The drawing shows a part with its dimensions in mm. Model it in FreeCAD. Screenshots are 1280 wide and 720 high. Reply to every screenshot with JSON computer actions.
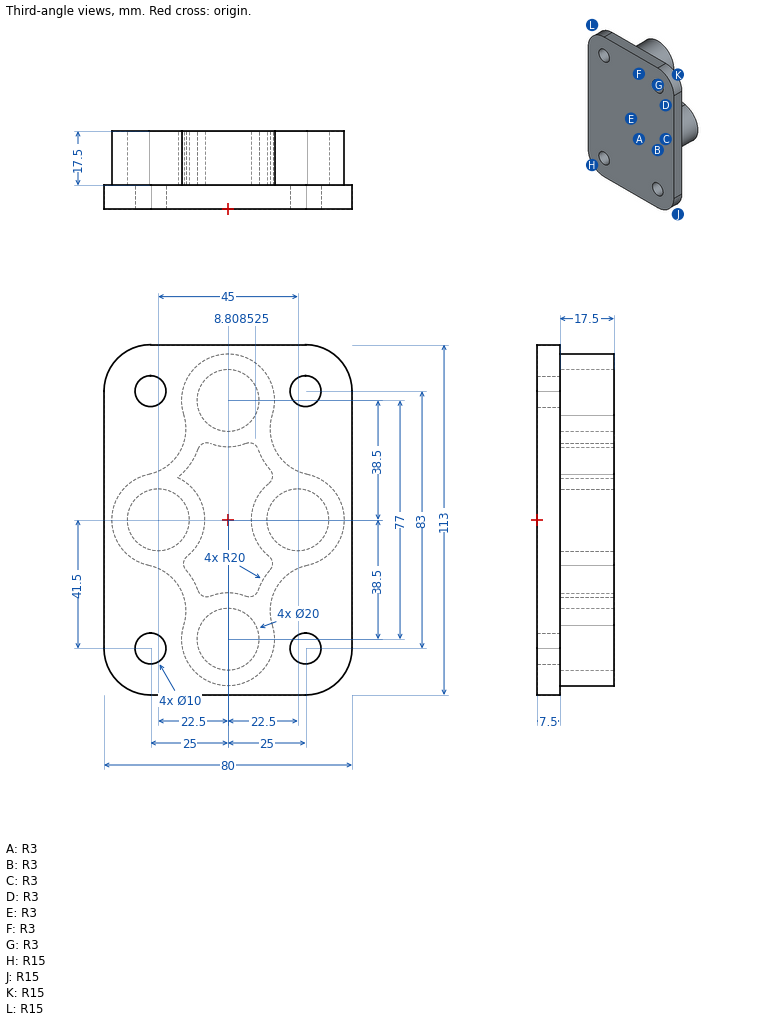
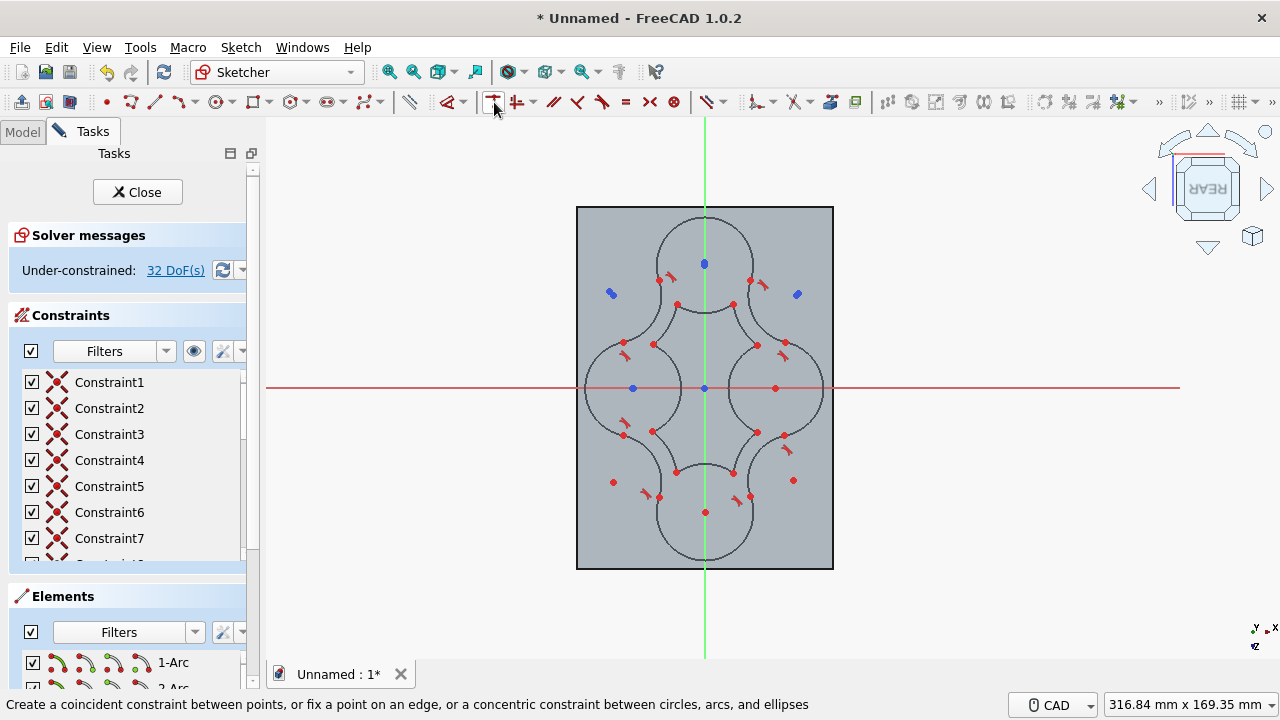
{"action": "left_click", "coordinate": [592, 364]}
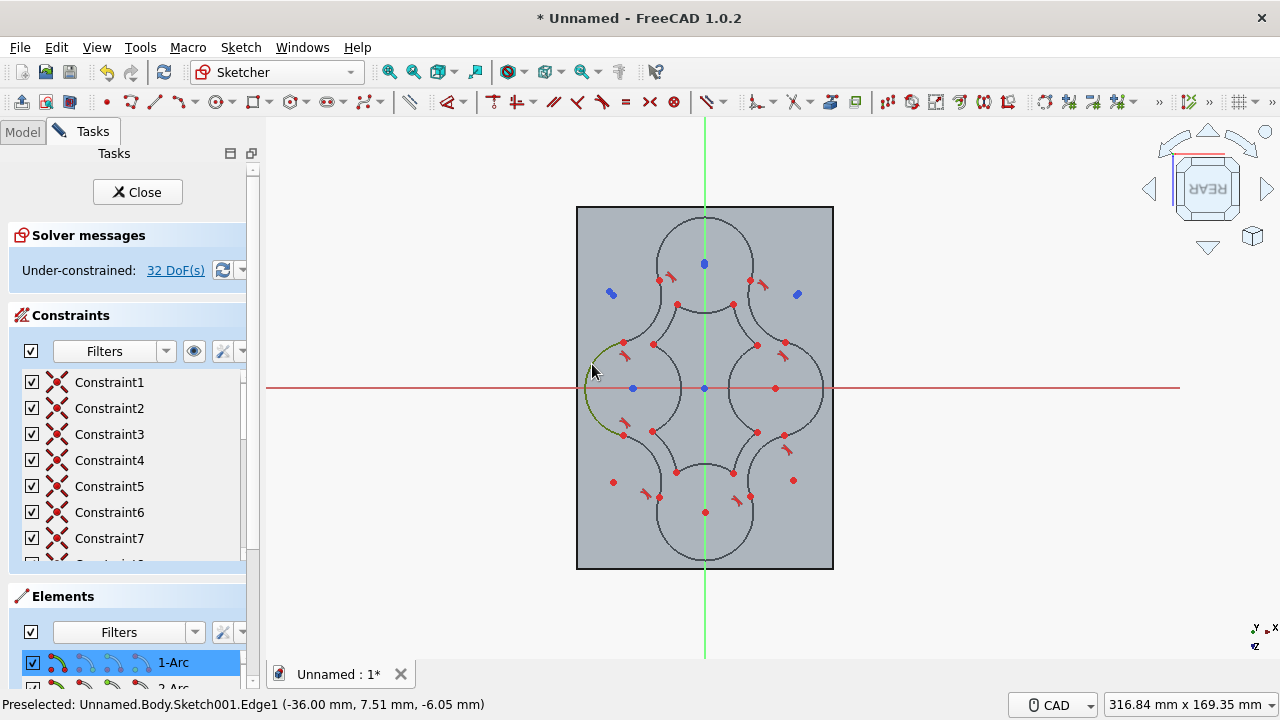
{"action": "left_click", "coordinate": [676, 410]}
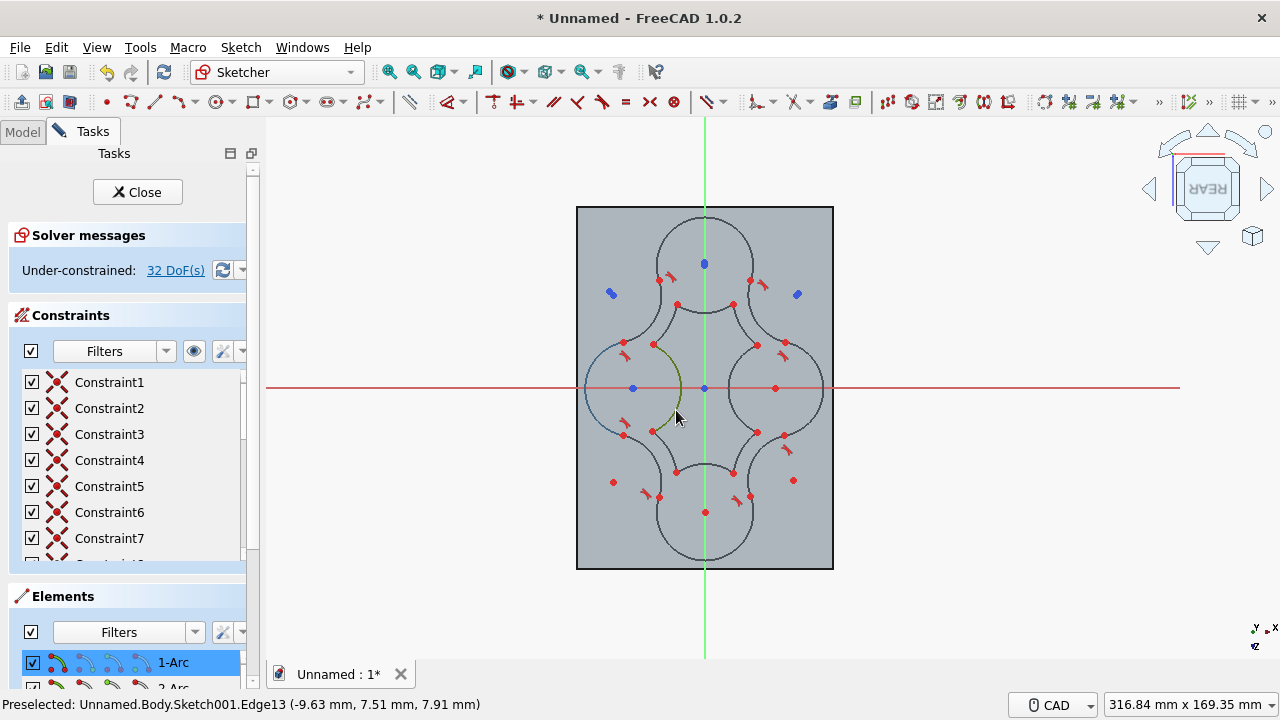
{"action": "left_click", "coordinate": [494, 102]}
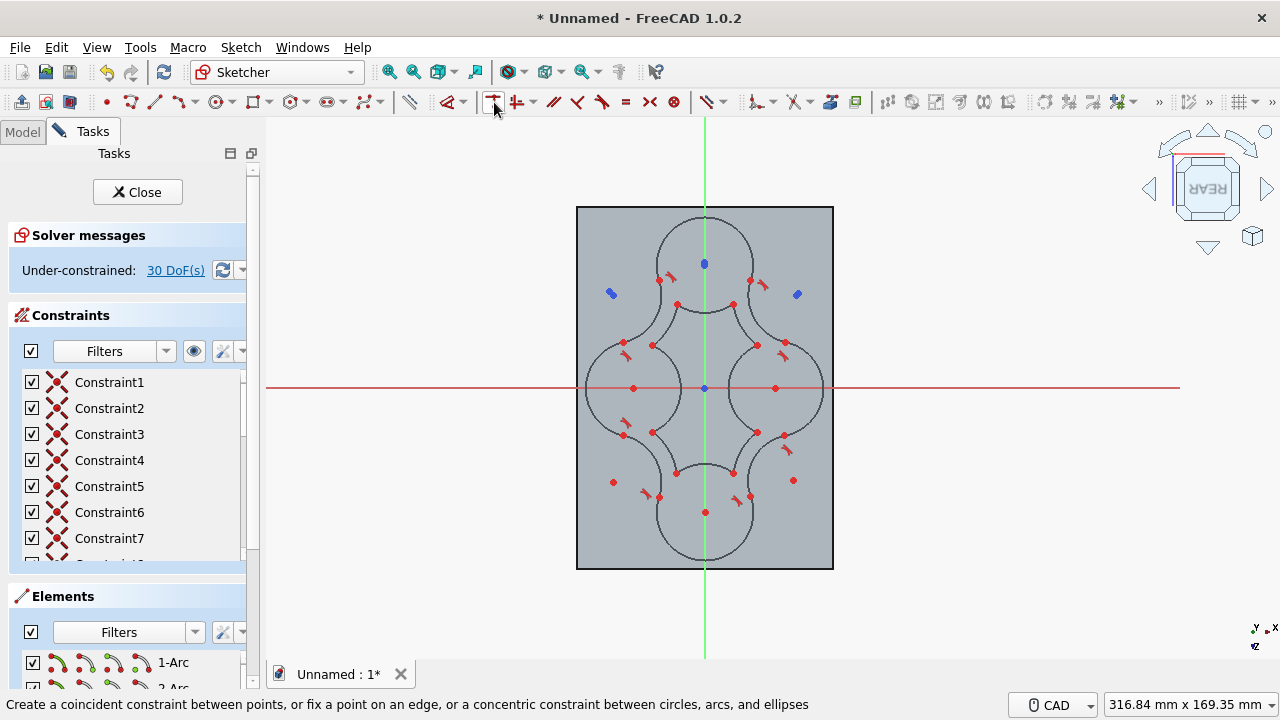
{"action": "left_click", "coordinate": [645, 332]}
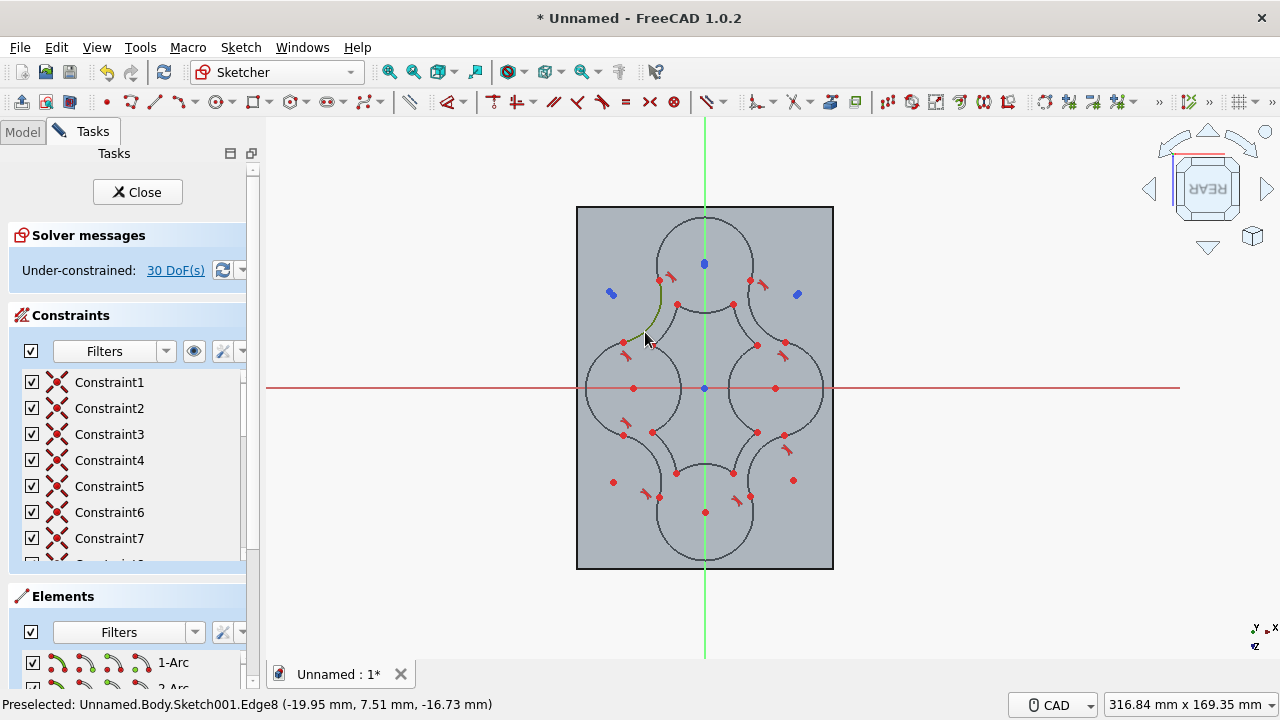
{"action": "left_click", "coordinate": [663, 336]}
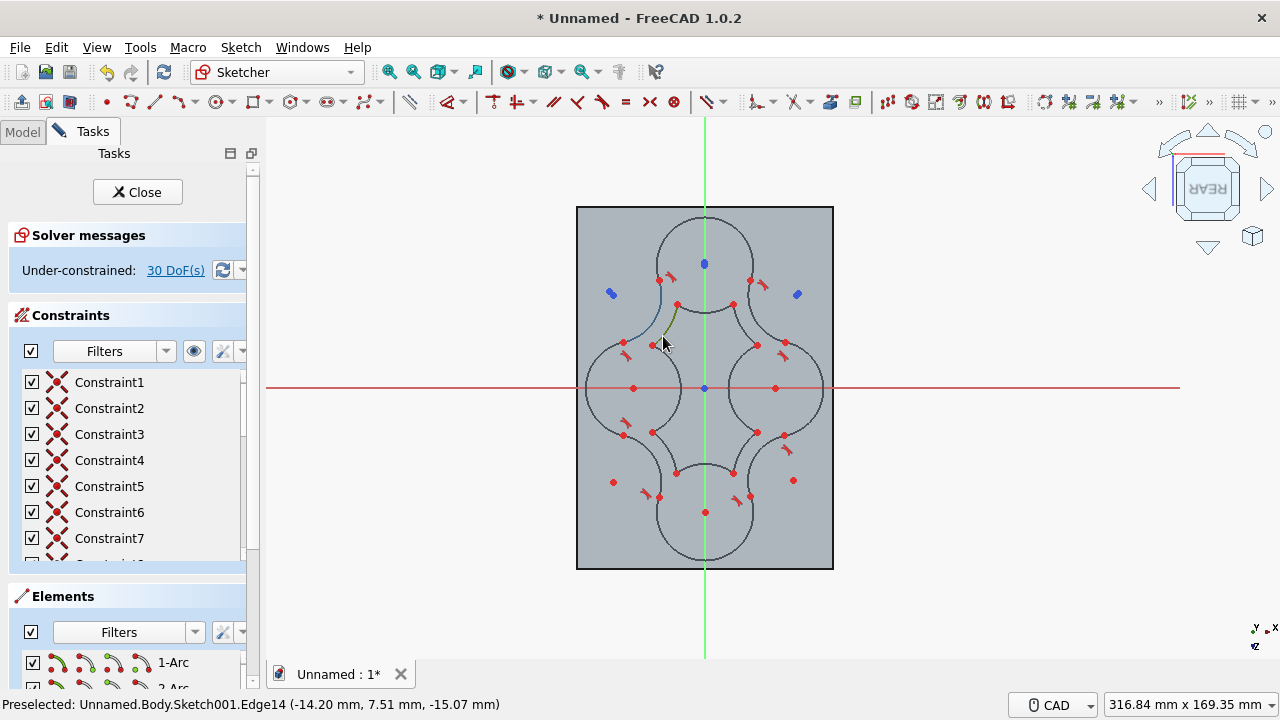
{"action": "key", "text": "c"}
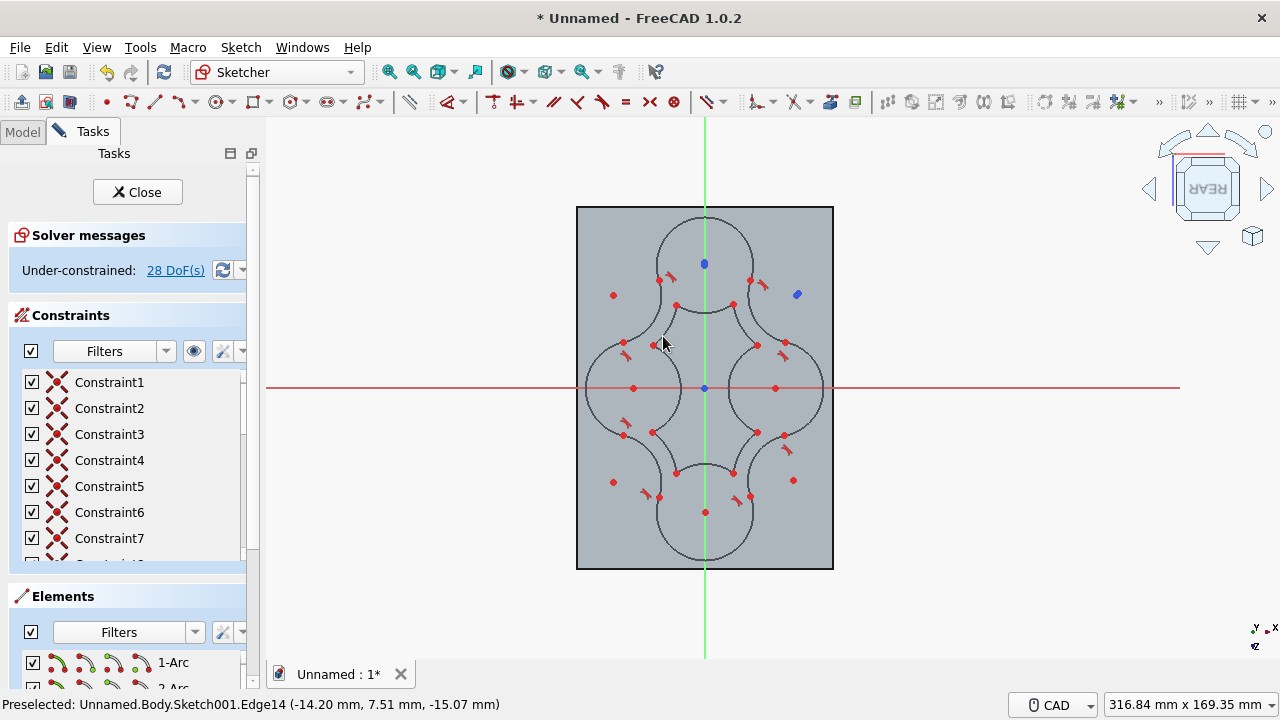
{"action": "left_click", "coordinate": [738, 231]}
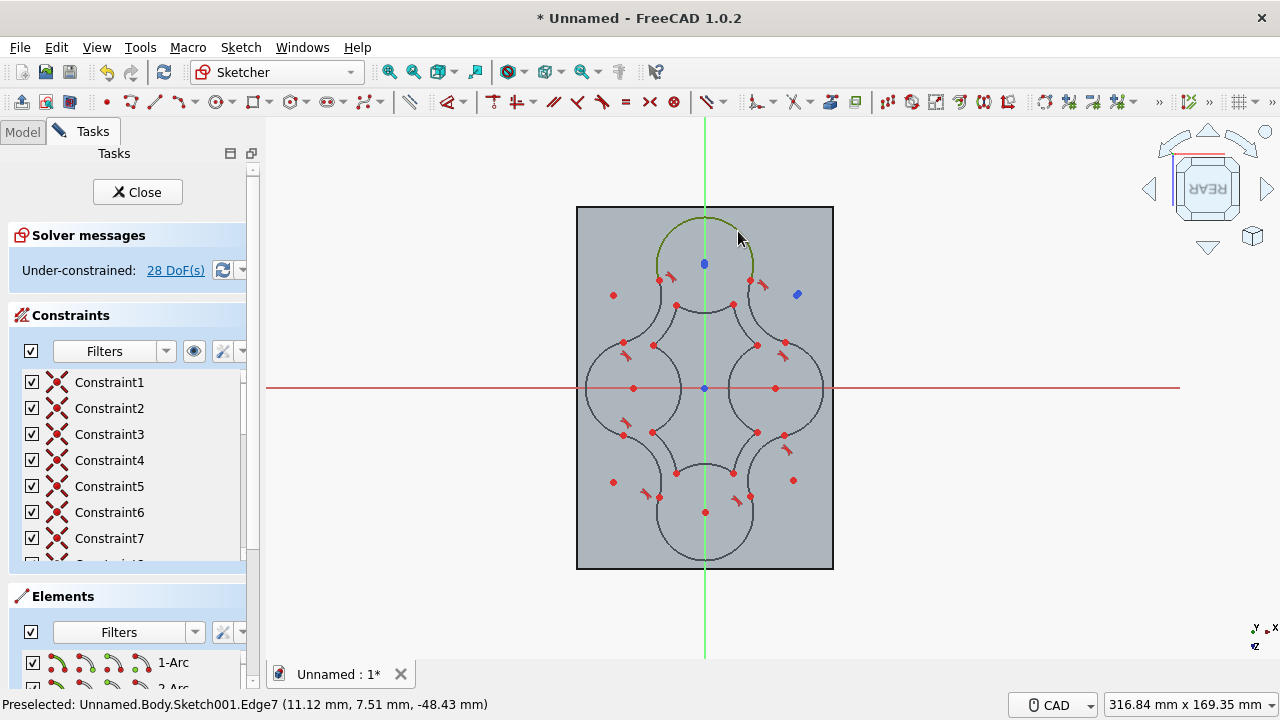
{"action": "left_click", "coordinate": [693, 312]}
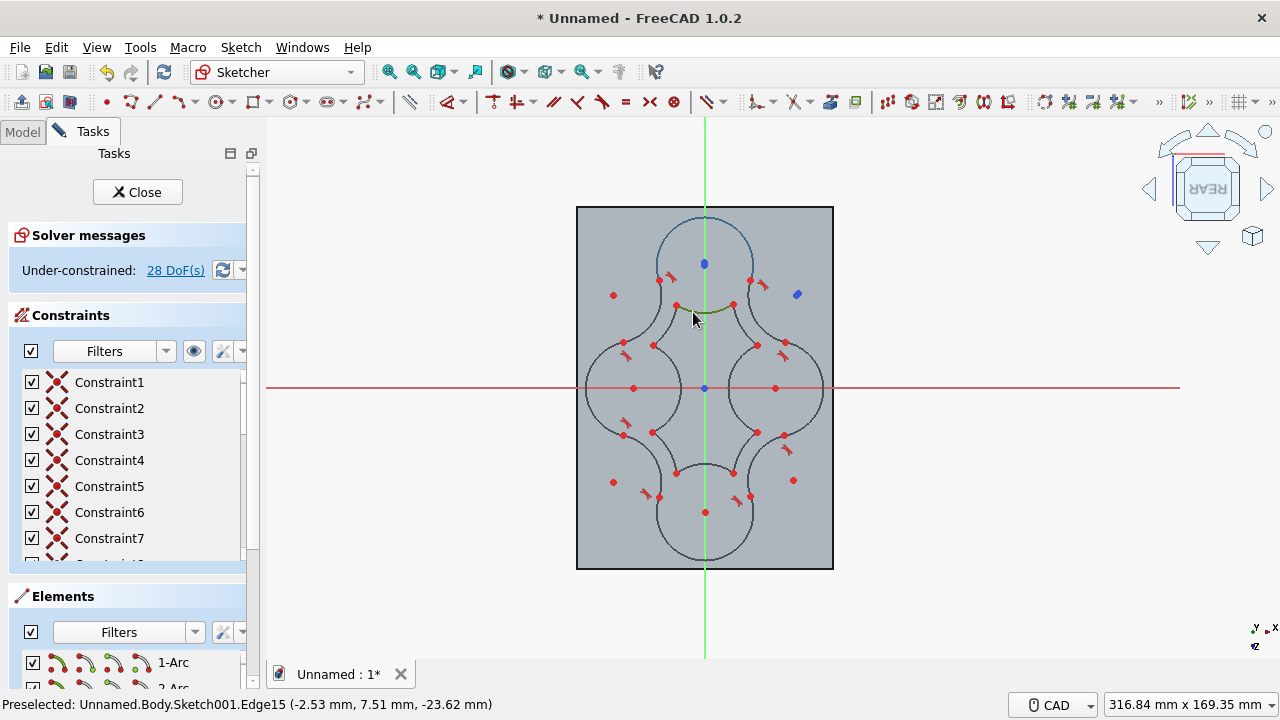
{"action": "left_click", "coordinate": [494, 102]}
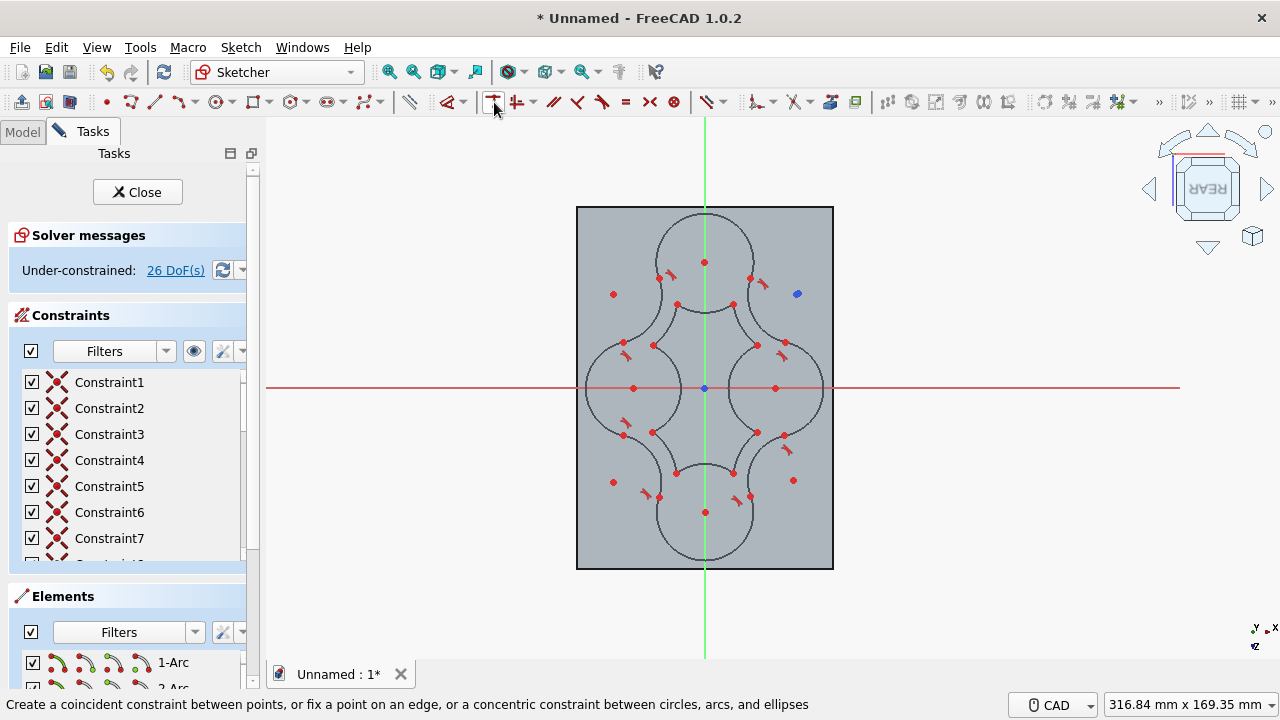
{"action": "left_click", "coordinate": [749, 303]}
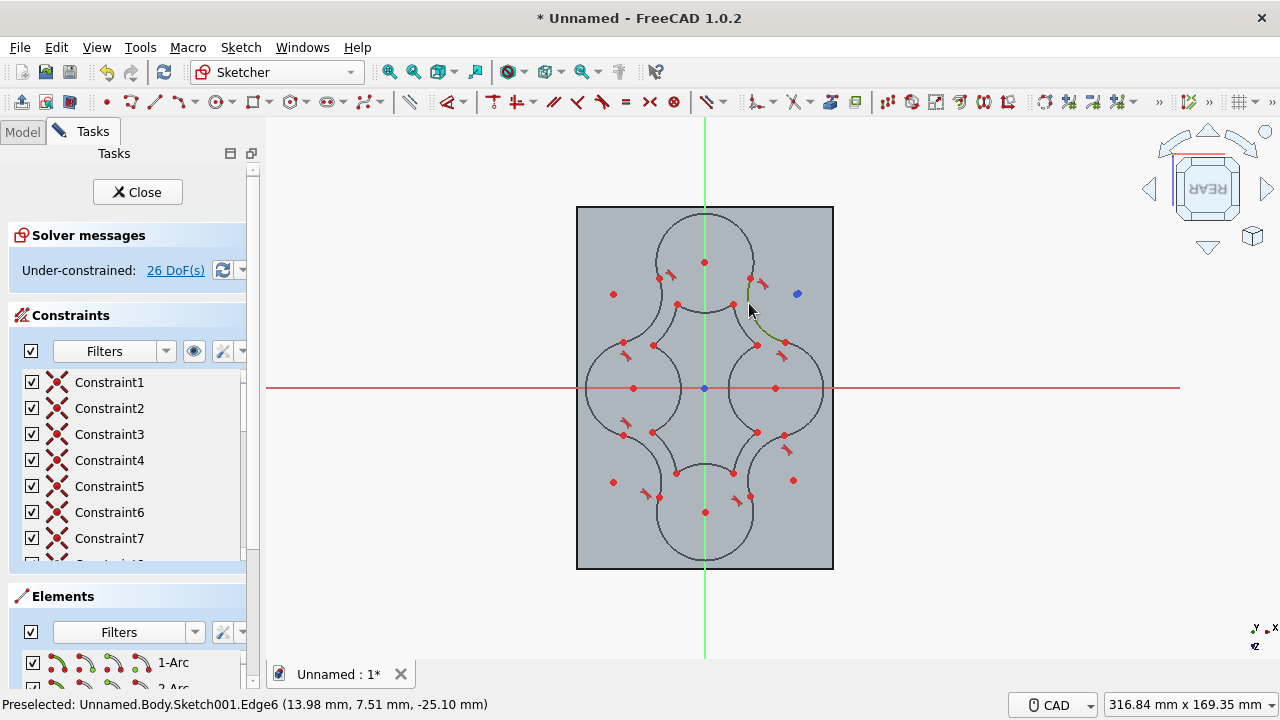
{"action": "left_click", "coordinate": [737, 318]}